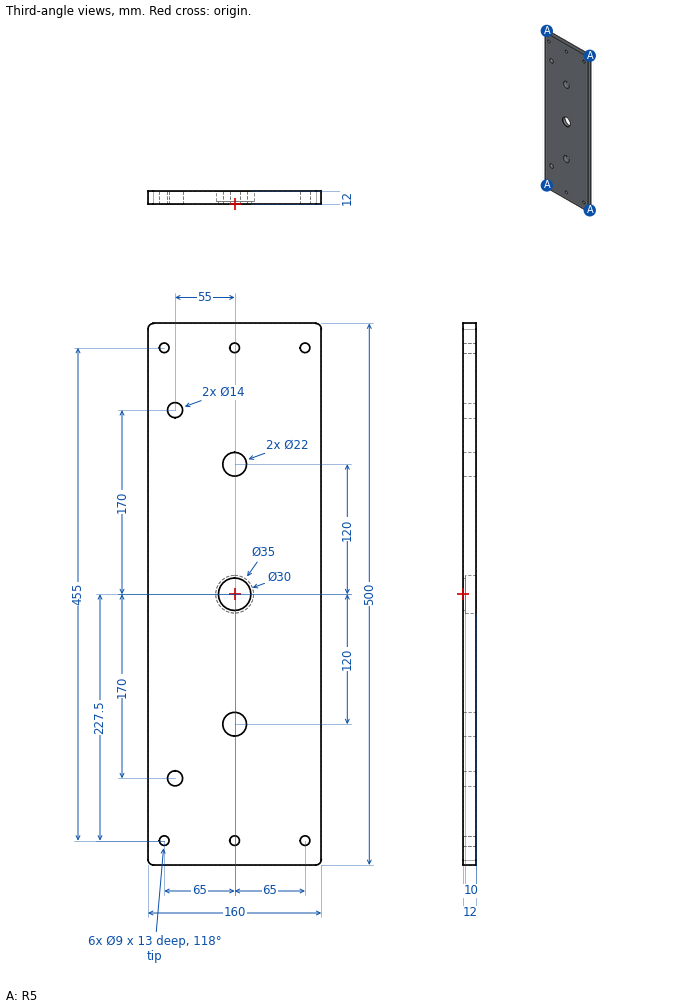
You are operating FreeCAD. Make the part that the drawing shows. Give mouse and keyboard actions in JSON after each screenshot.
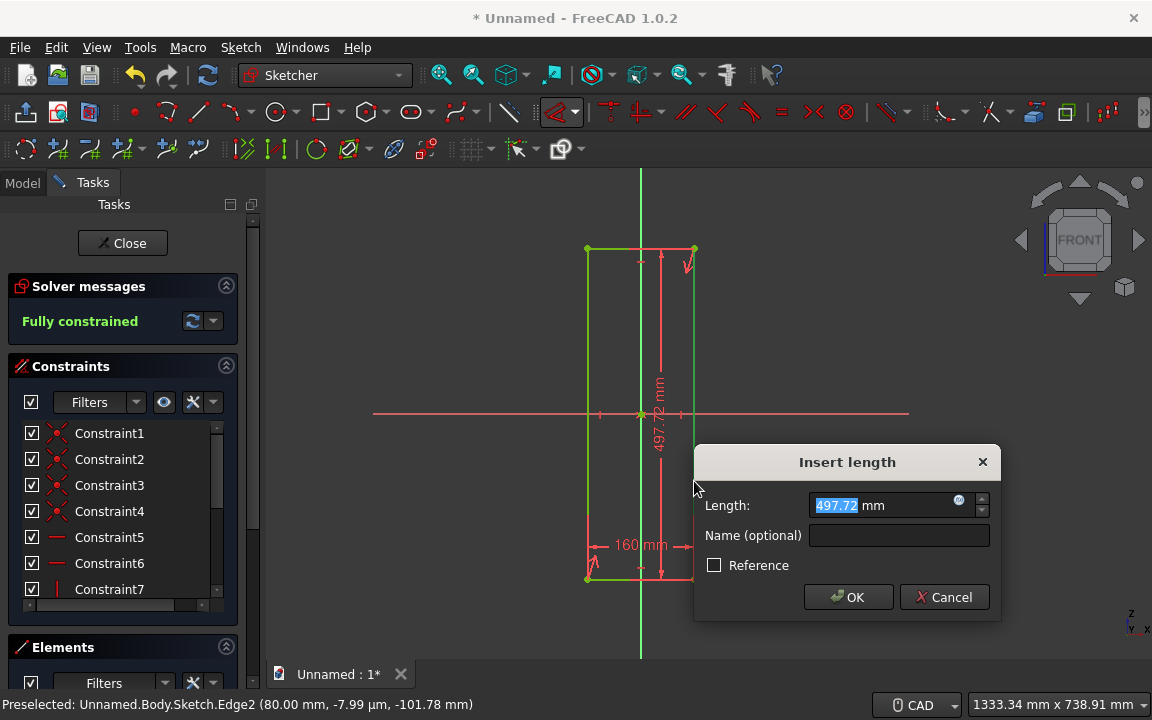
{"action": "type", "text": "500"}
{"action": "key", "text": "Return"}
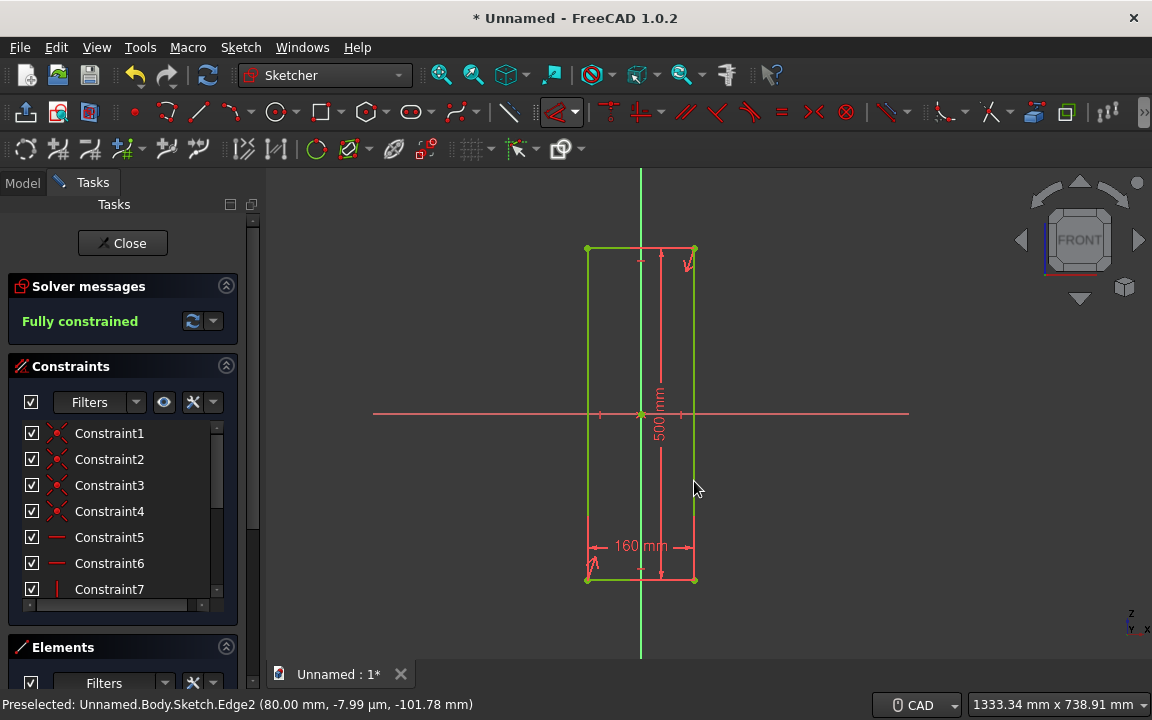
{"action": "left_click", "coordinate": [123, 243]}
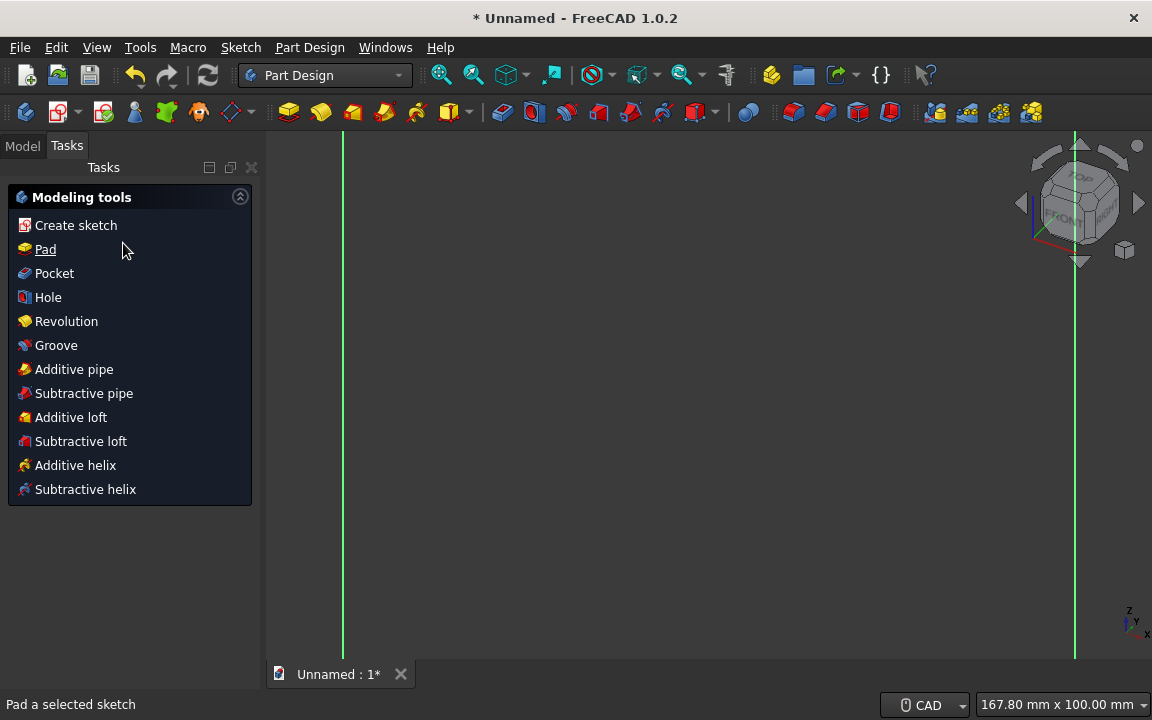
{"action": "left_click", "coordinate": [290, 112]}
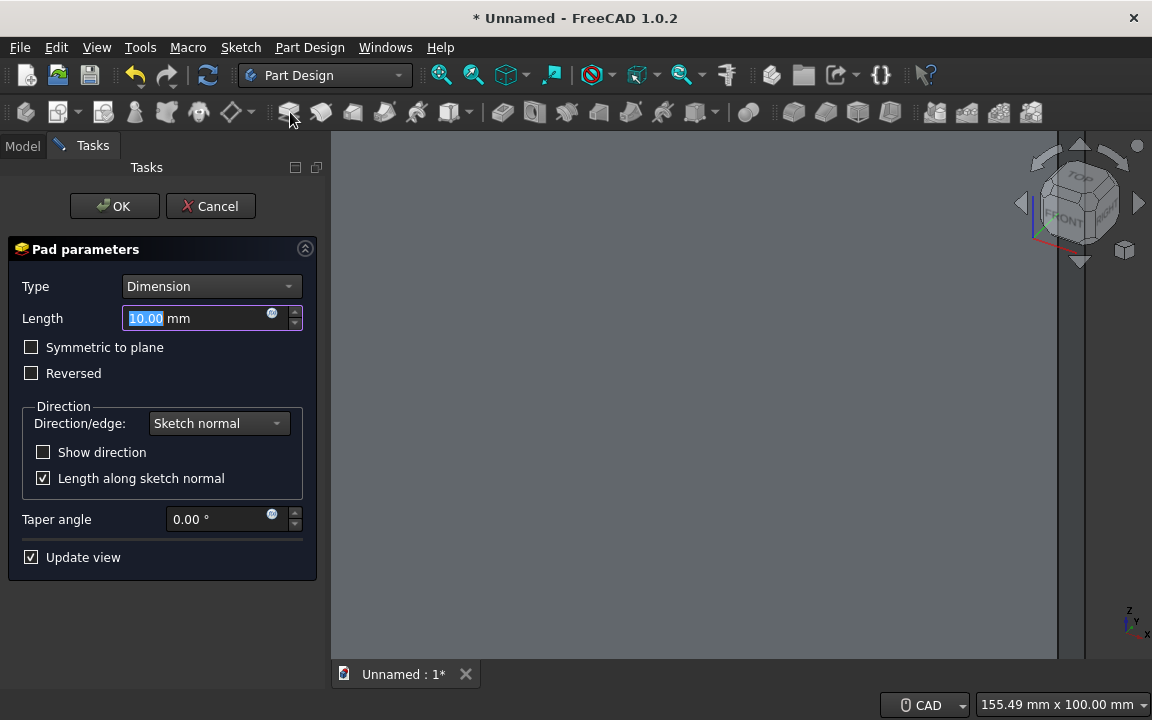
{"action": "type", "text": "12"}
{"action": "key", "text": "Tab"}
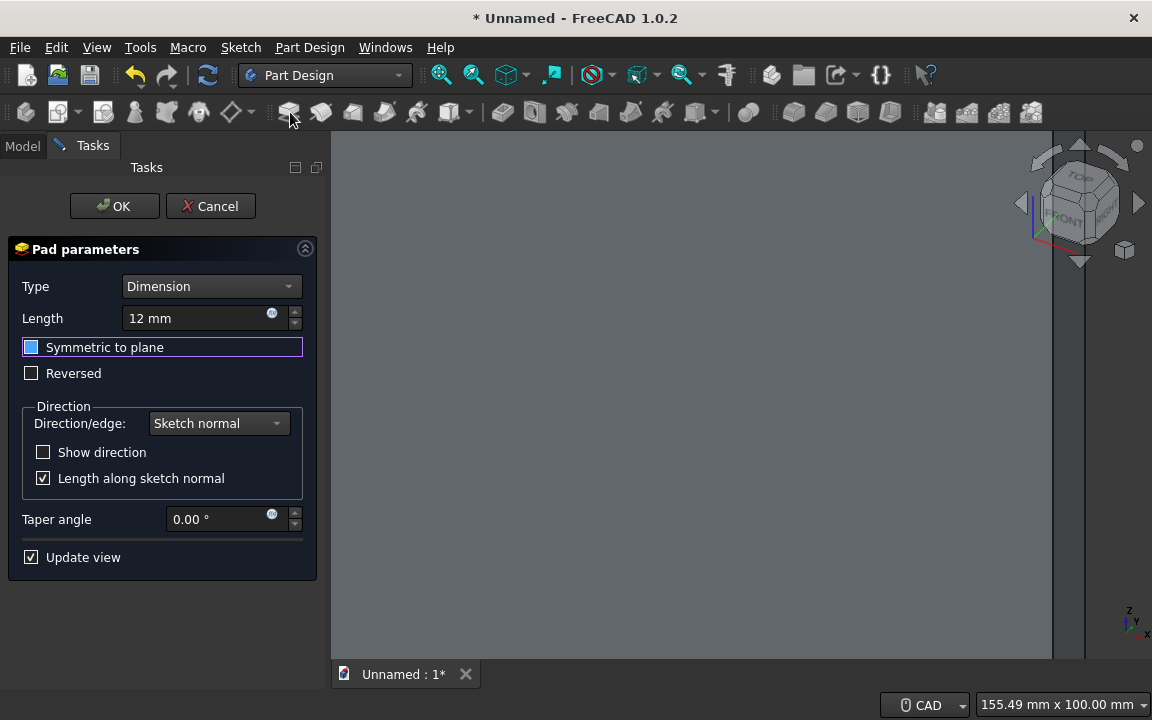
{"action": "left_click", "coordinate": [30, 373]}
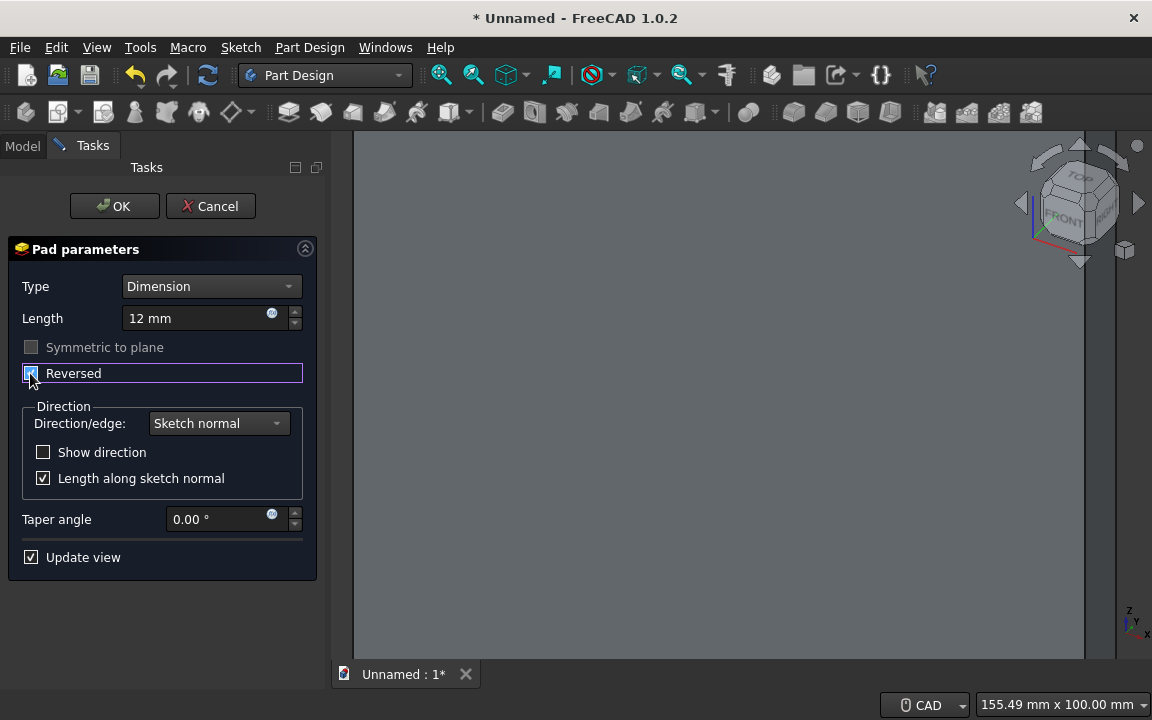
{"action": "left_click", "coordinate": [115, 206]}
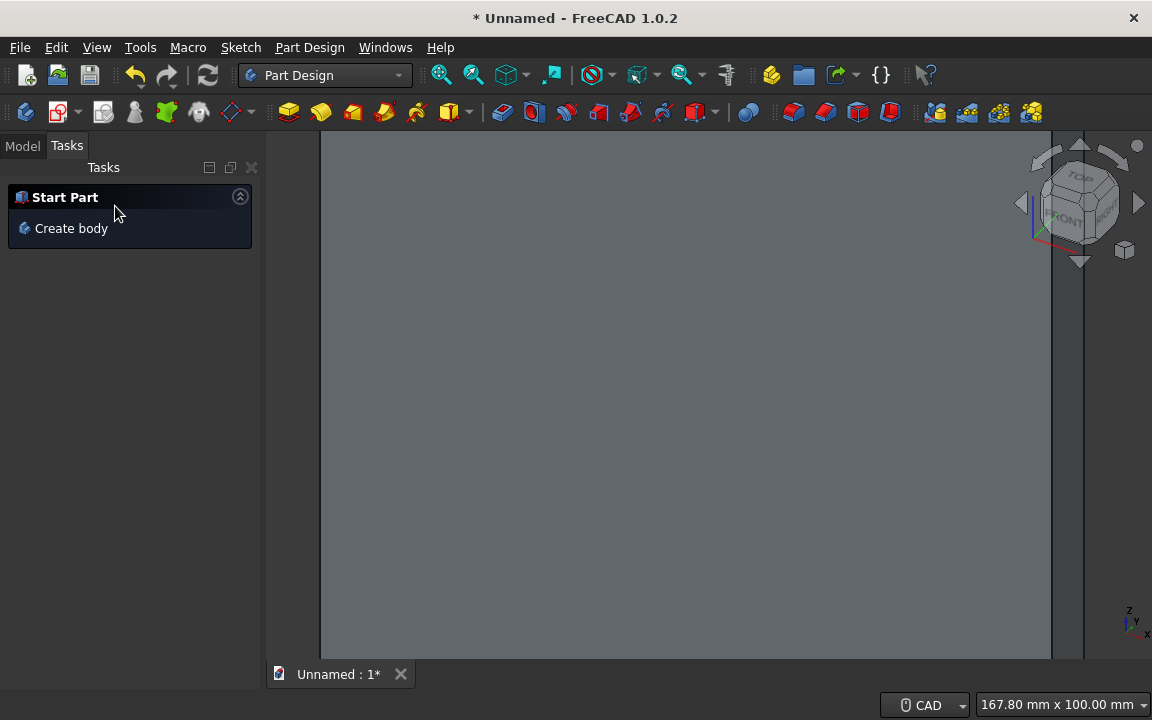
{"action": "left_click", "coordinate": [442, 76]}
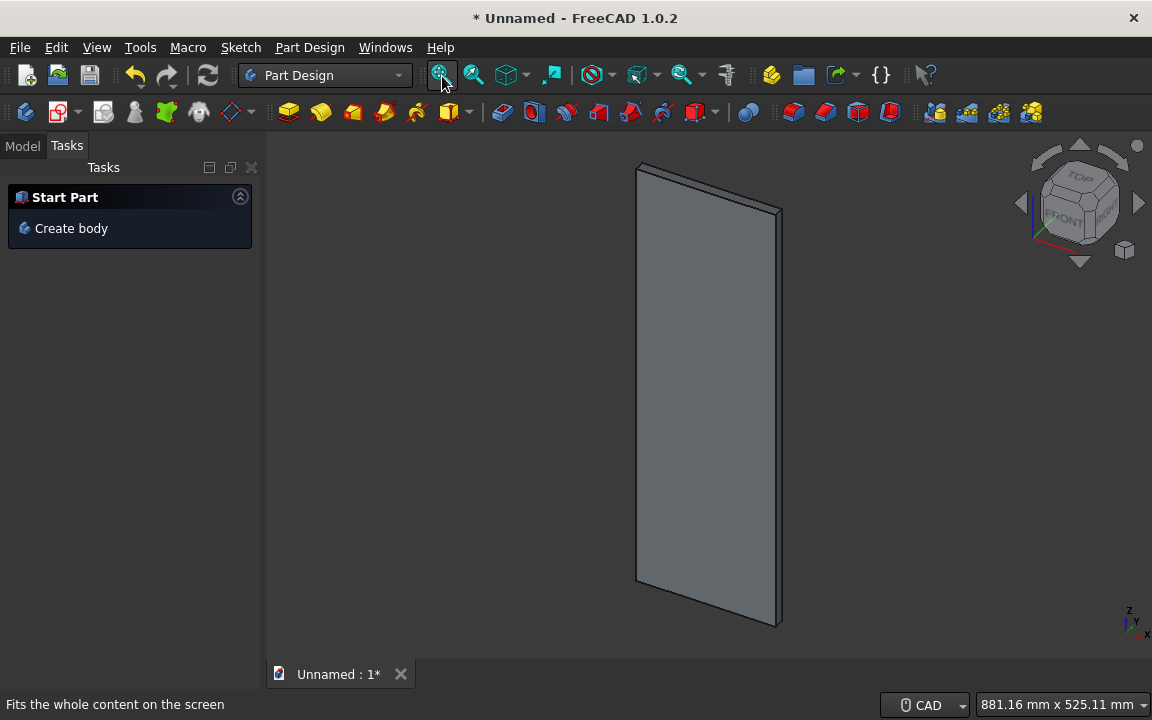
{"action": "key", "text": "4"}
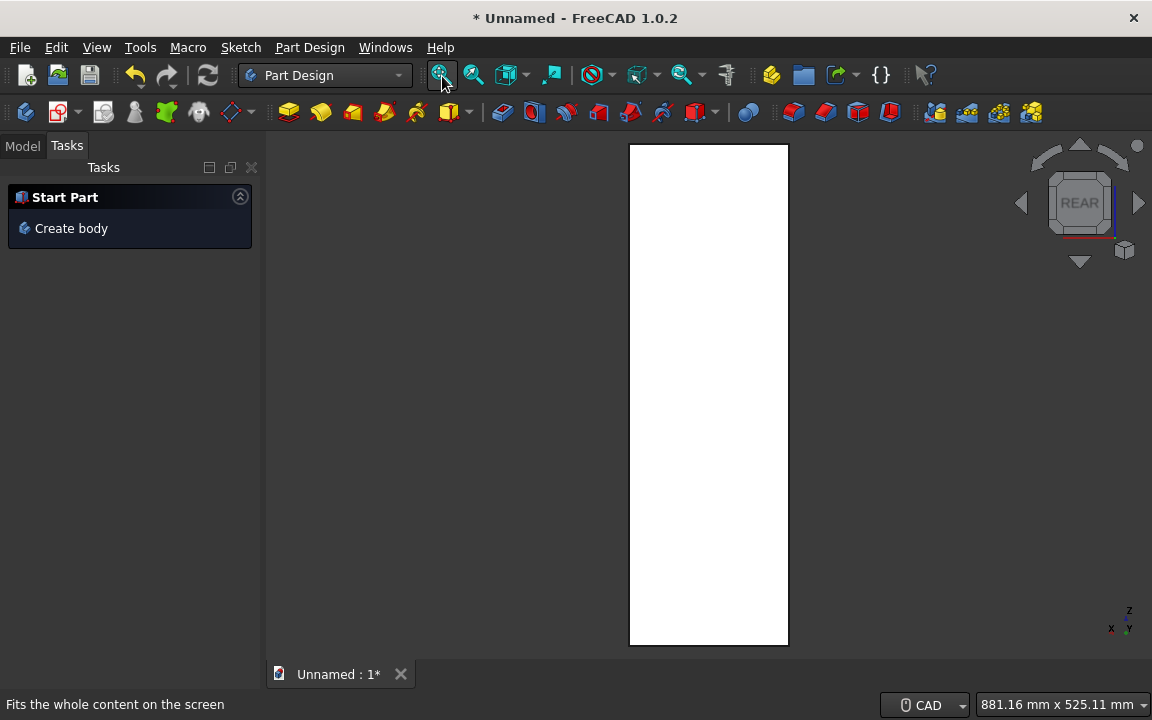
{"action": "left_click", "coordinate": [709, 250]}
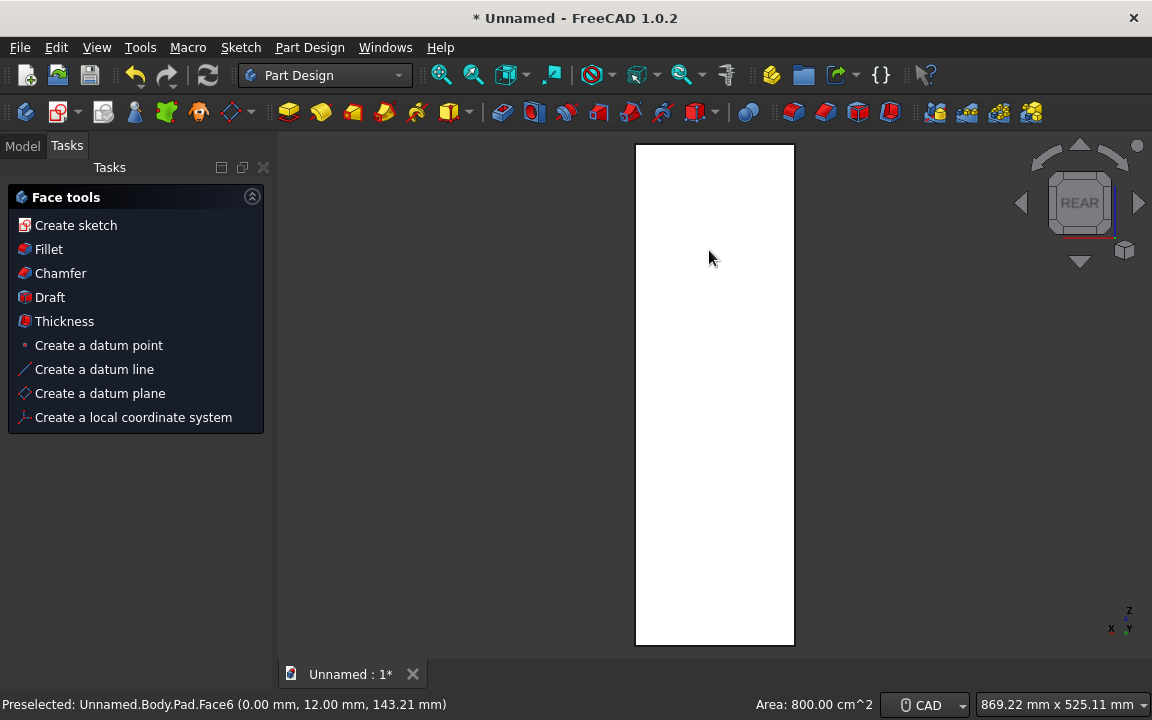
{"action": "left_click", "coordinate": [58, 112]}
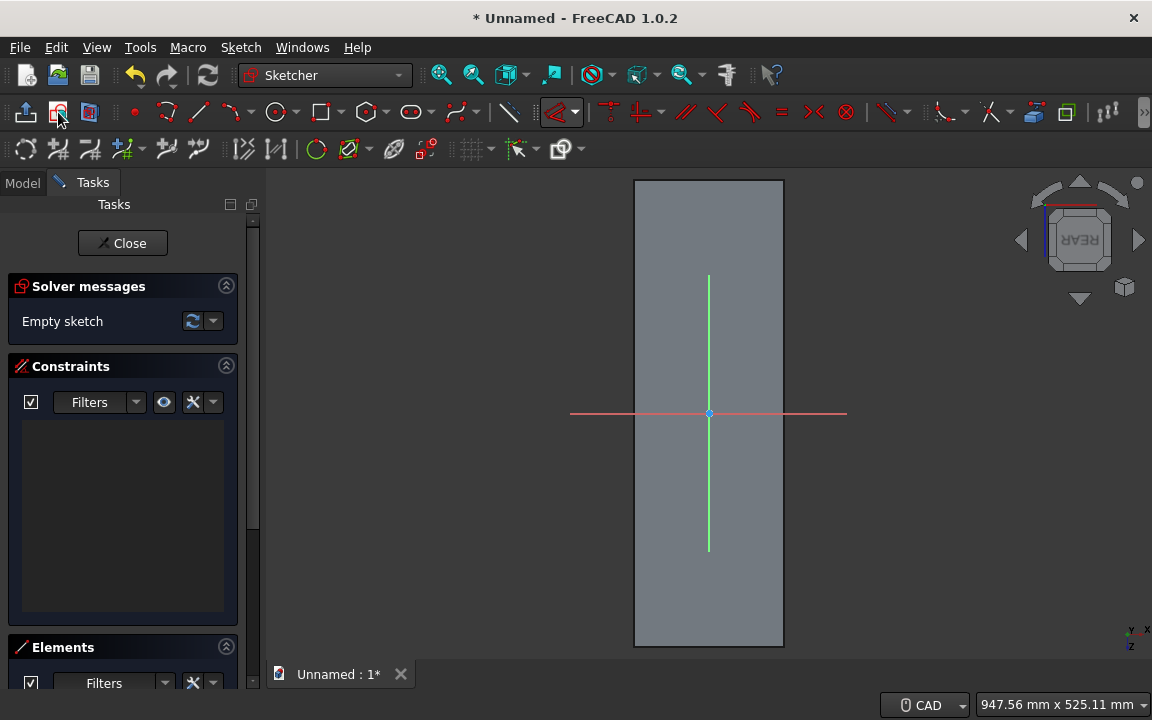
{"action": "left_click", "coordinate": [276, 112]}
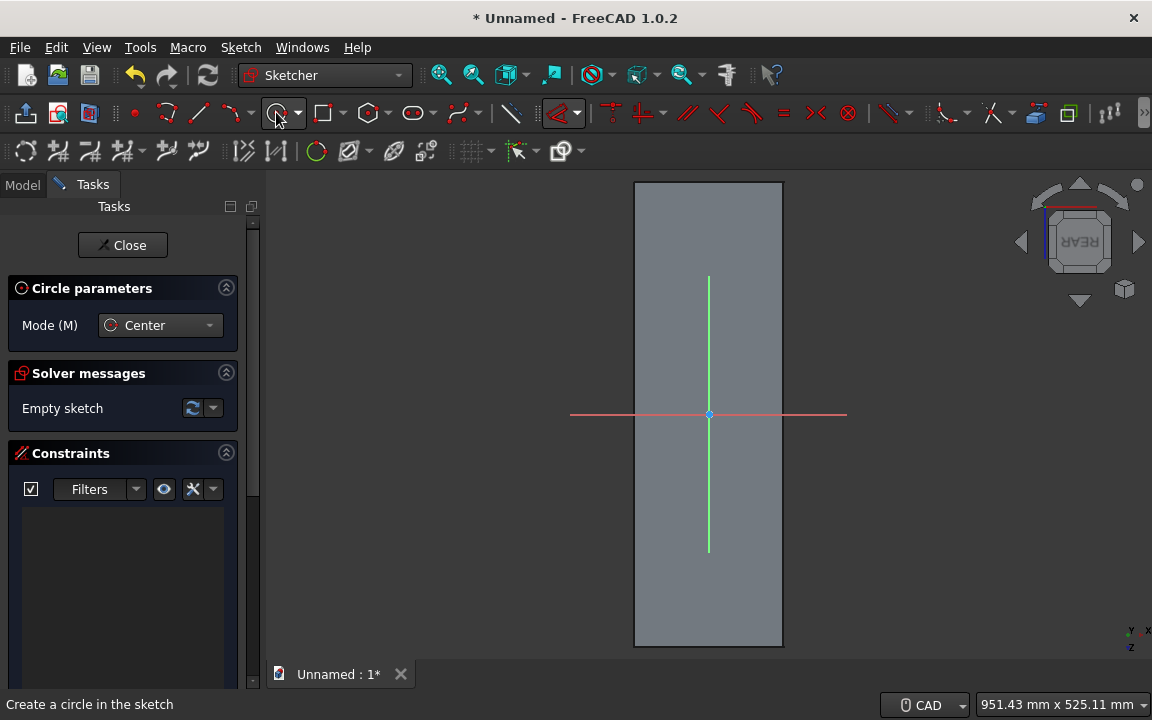
{"action": "scroll", "coordinate": [709, 415], "scroll_direction": "up", "scroll_amount": 3}